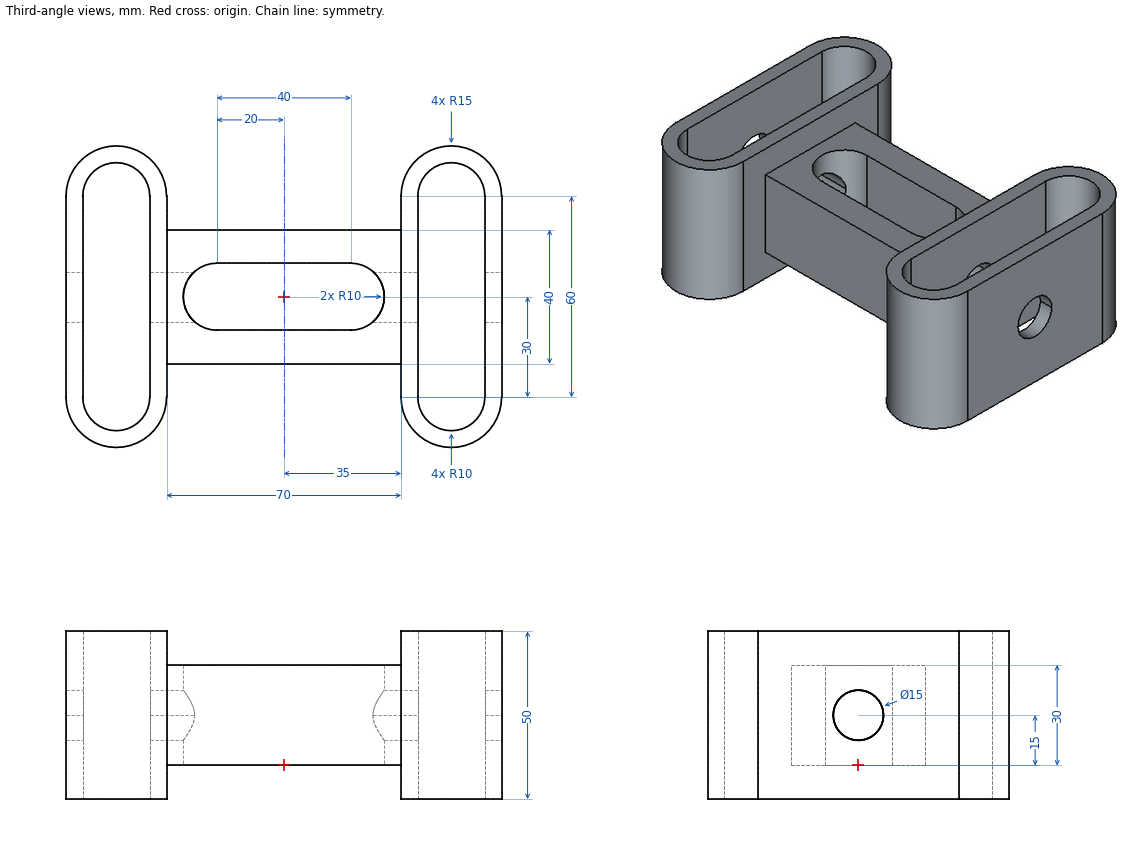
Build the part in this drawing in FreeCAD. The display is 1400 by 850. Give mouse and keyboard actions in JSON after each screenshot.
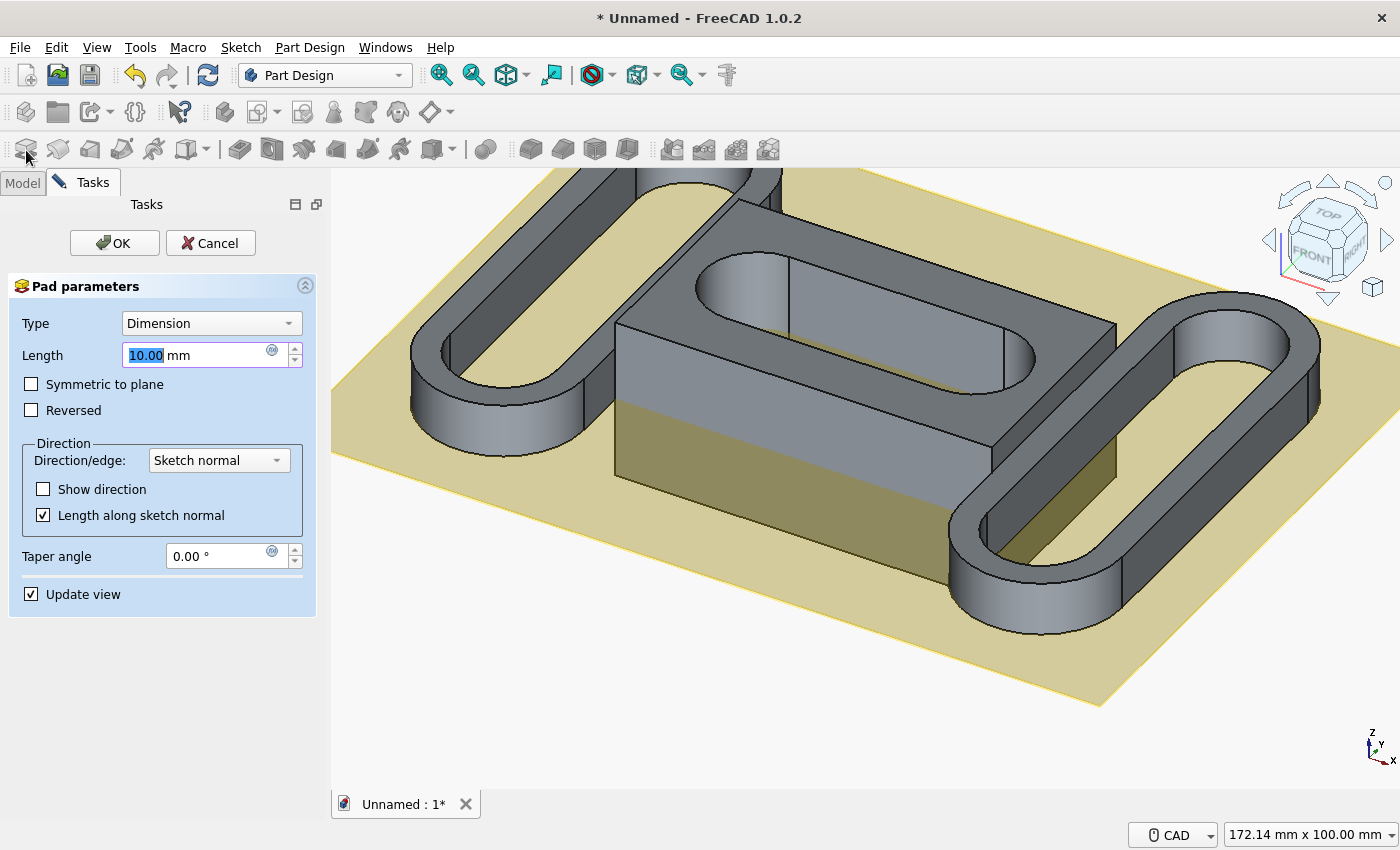
{"action": "type", "text": "50"}
{"action": "key", "text": "Tab"}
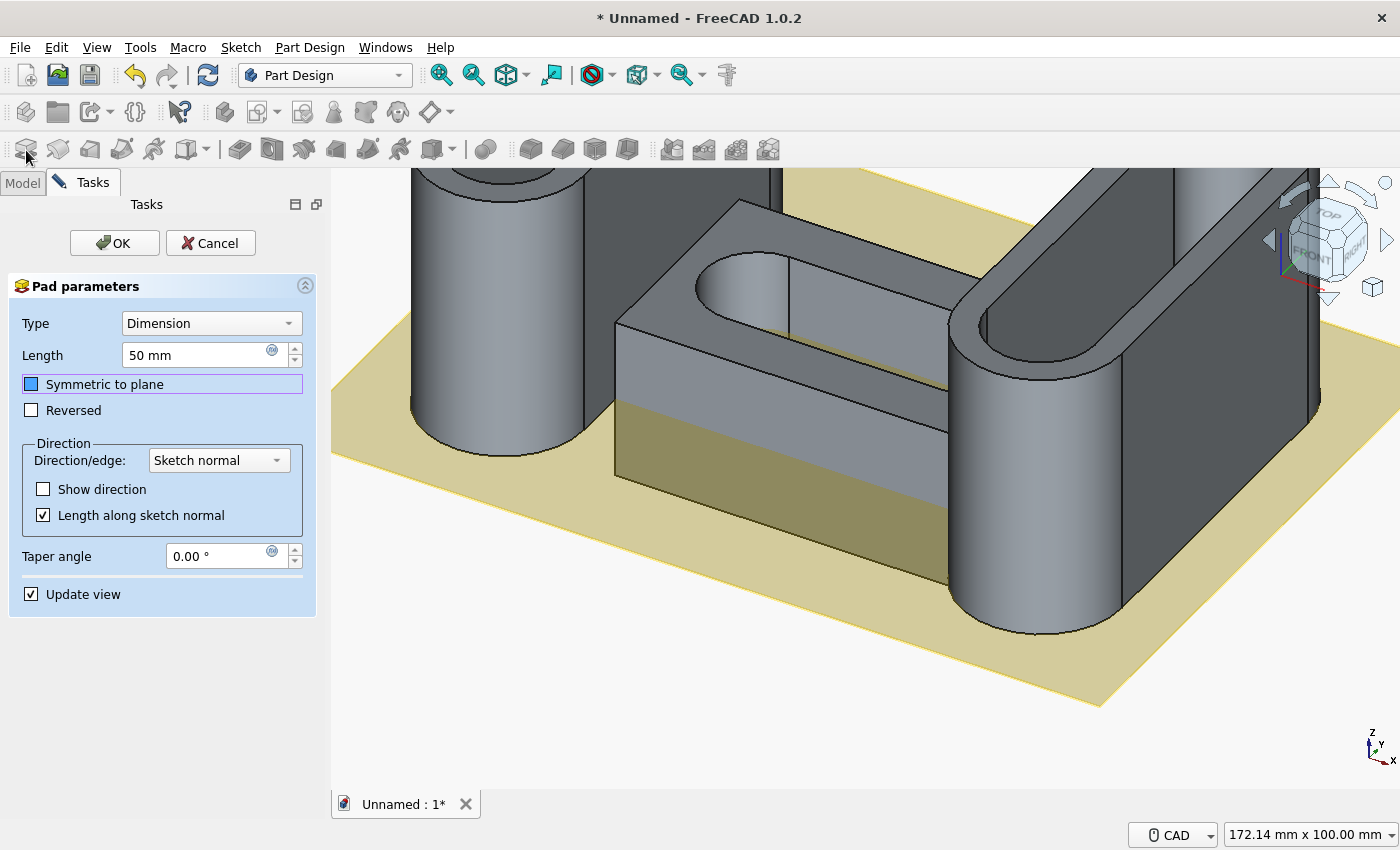
{"action": "left_click", "coordinate": [30, 384]}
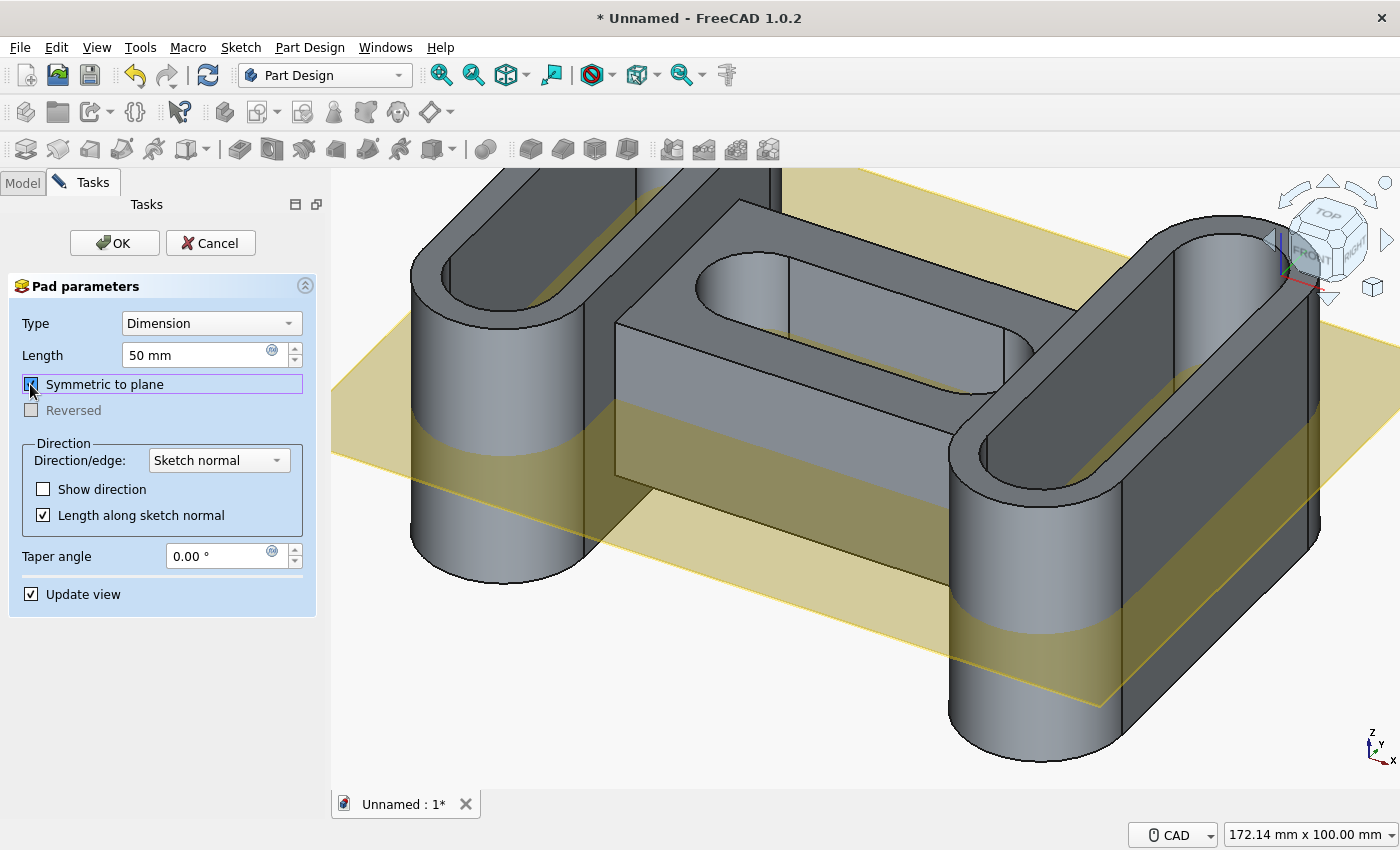
{"action": "left_click", "coordinate": [115, 243]}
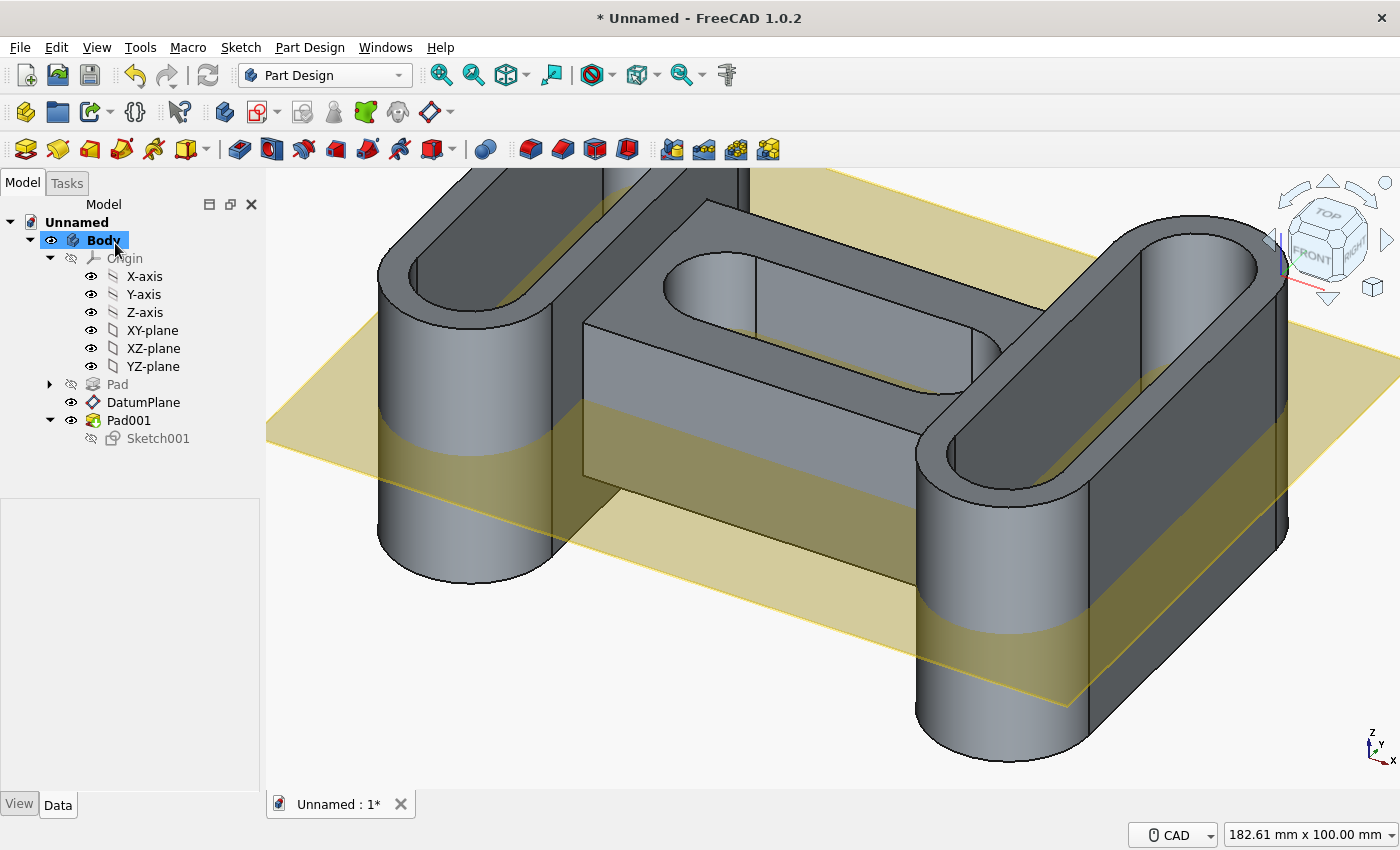
{"action": "left_click", "coordinate": [116, 402]}
{"action": "key", "text": "space"}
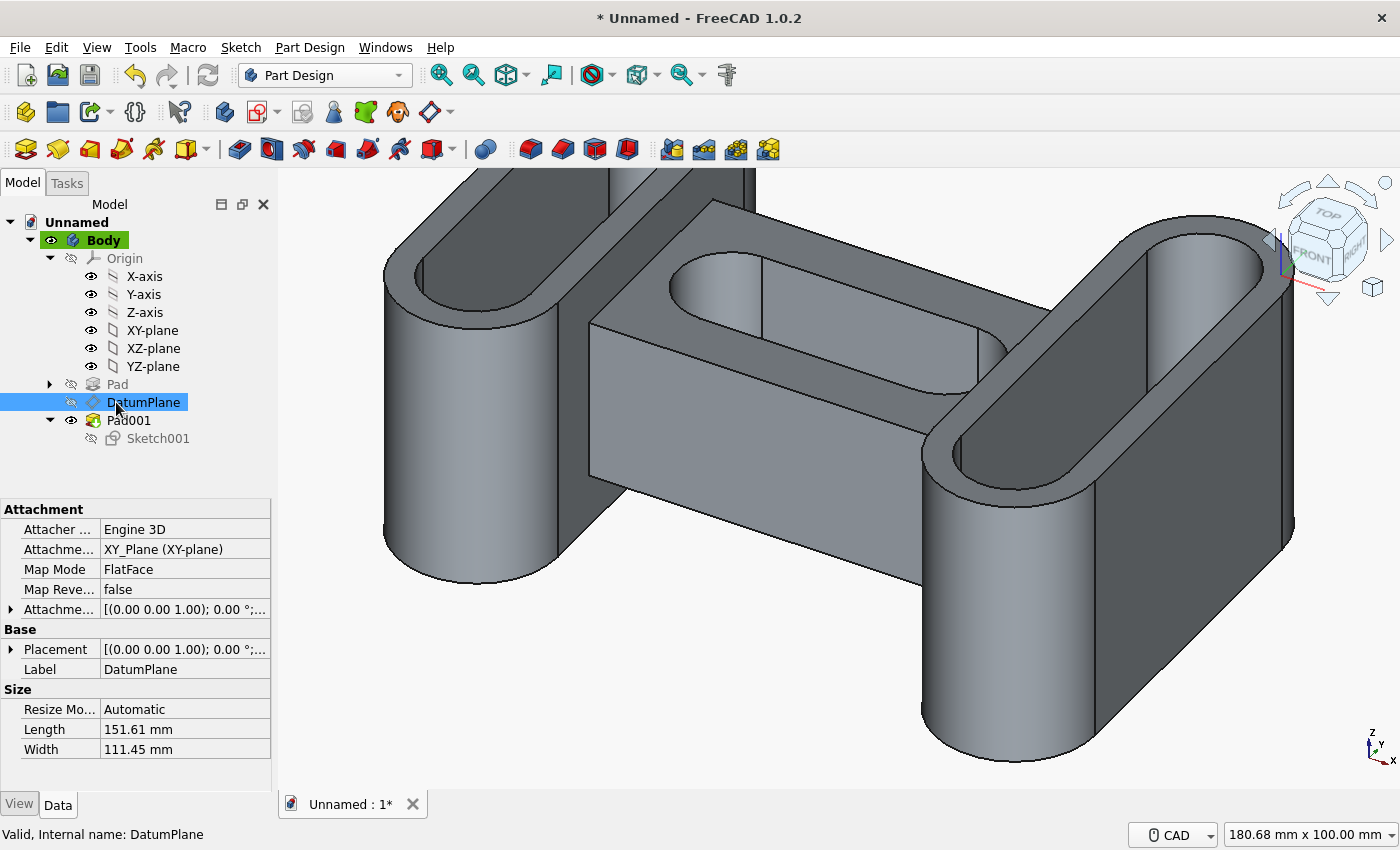
{"action": "key", "text": "v f"}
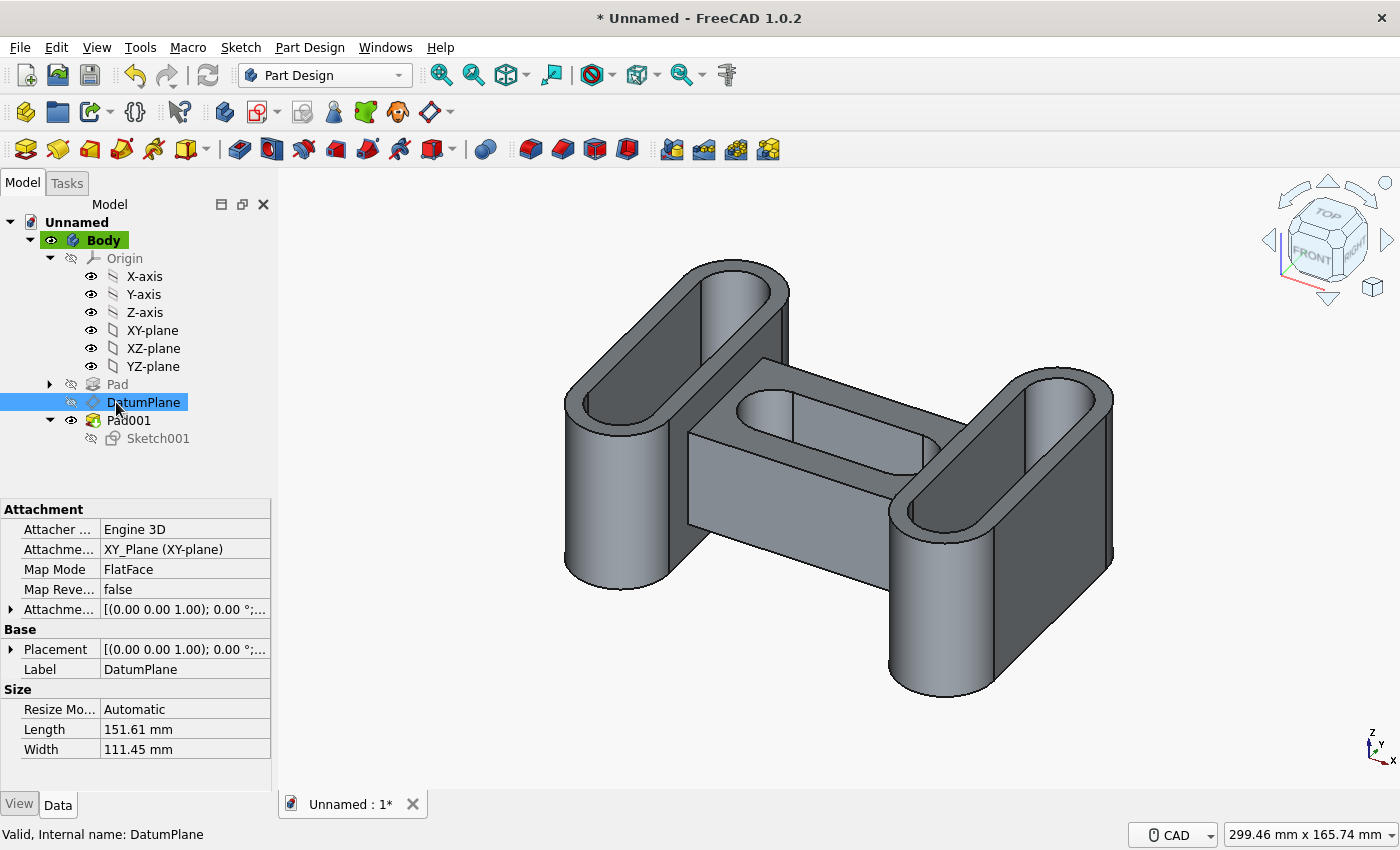
{"action": "left_click", "coordinate": [318, 749]}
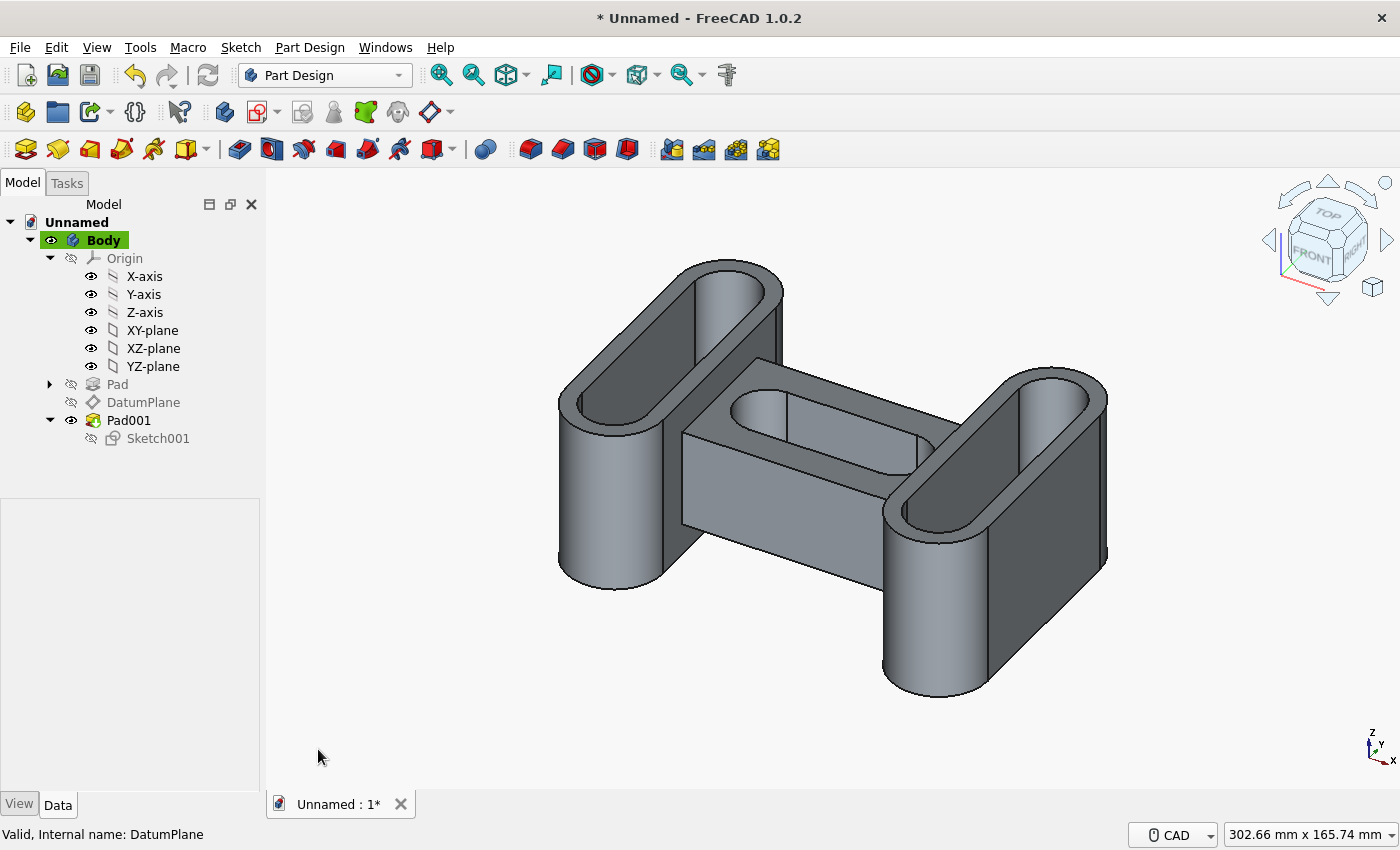
{"action": "left_click", "coordinate": [258, 112]}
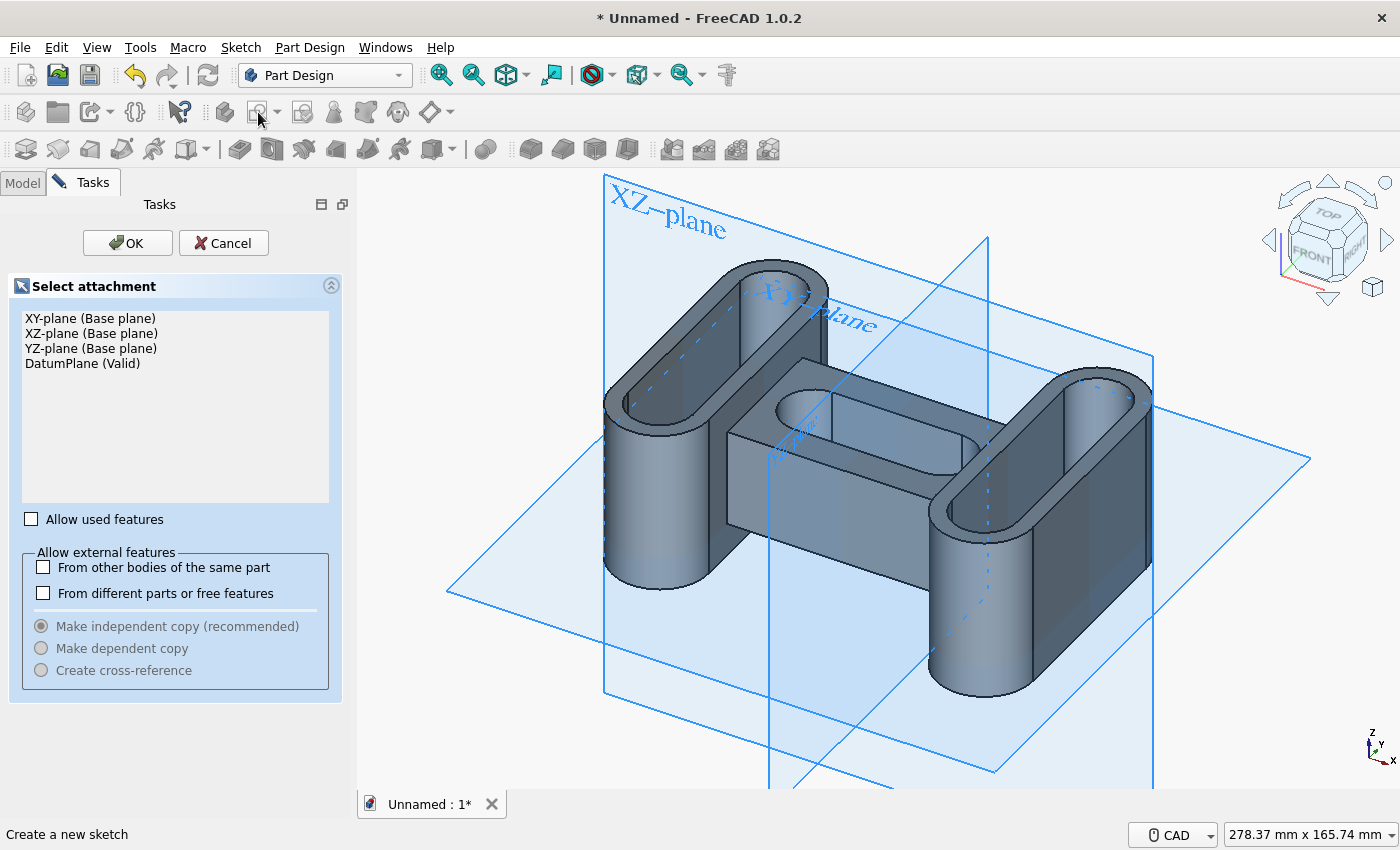
{"action": "left_click", "coordinate": [82, 348]}